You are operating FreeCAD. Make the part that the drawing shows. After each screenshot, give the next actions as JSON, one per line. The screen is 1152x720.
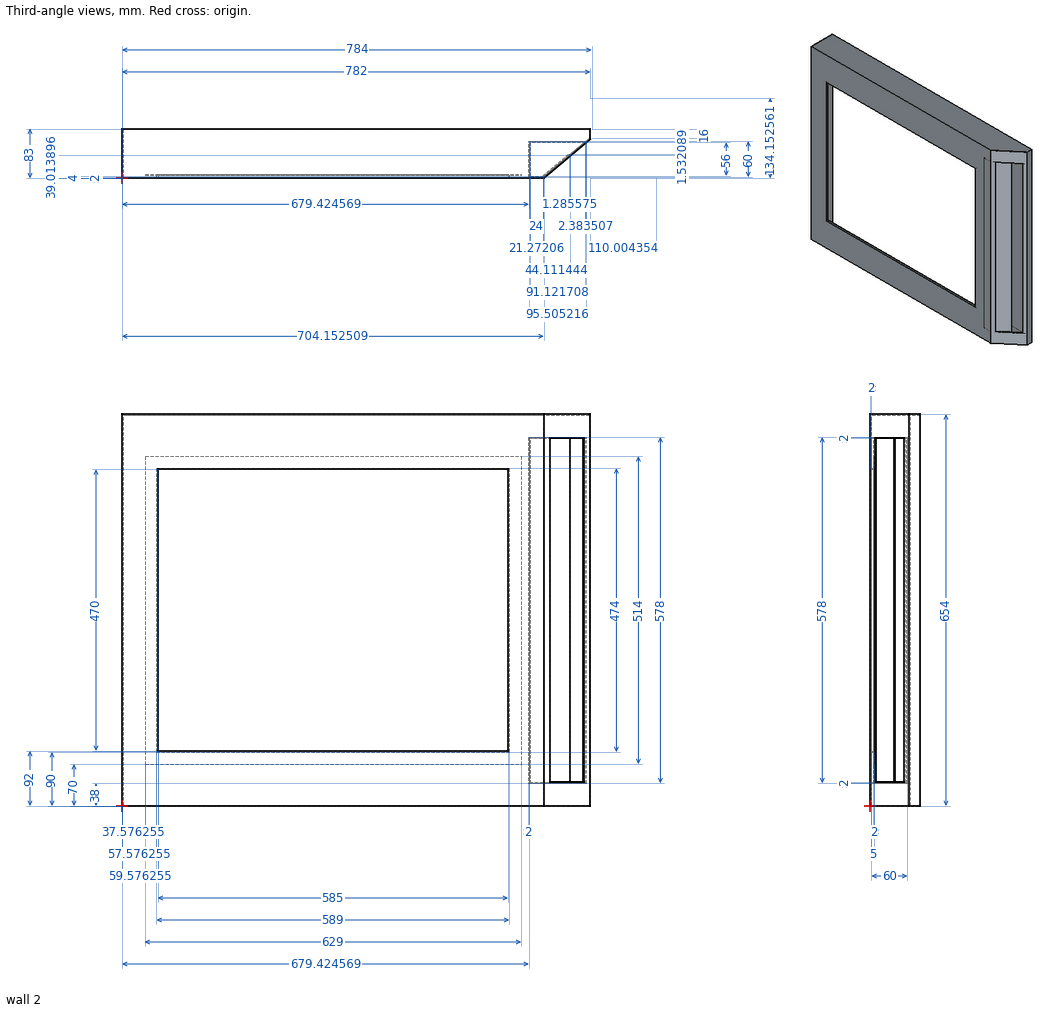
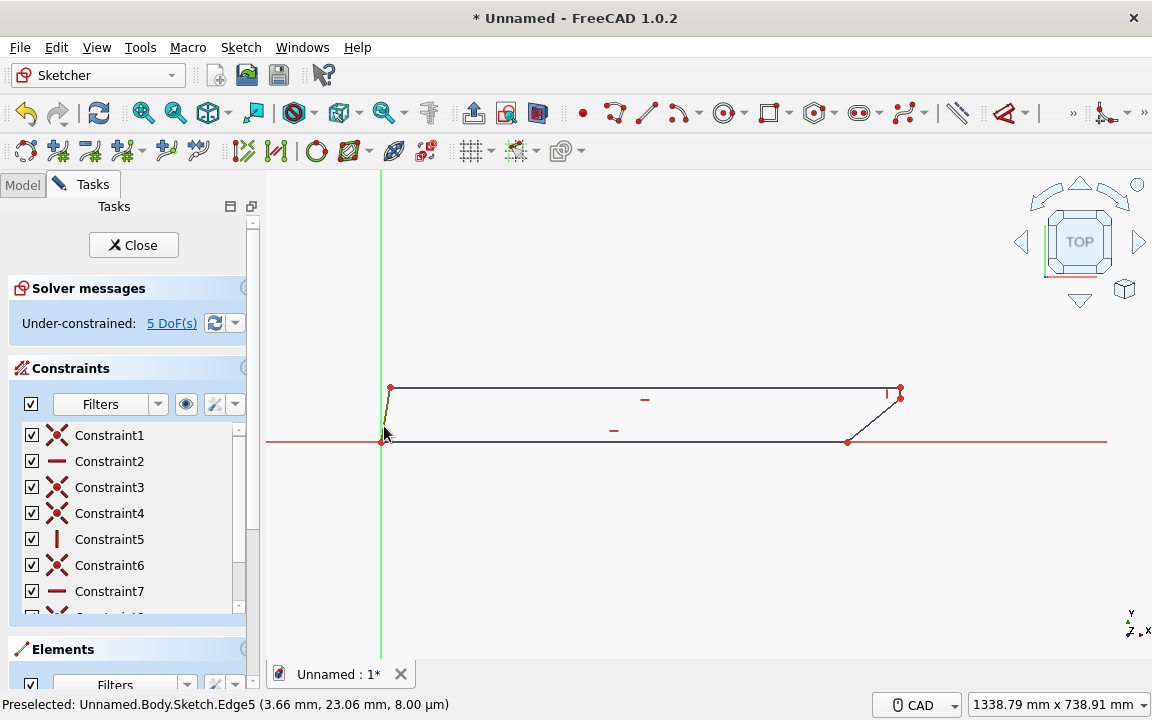
{"action": "key", "text": "v"}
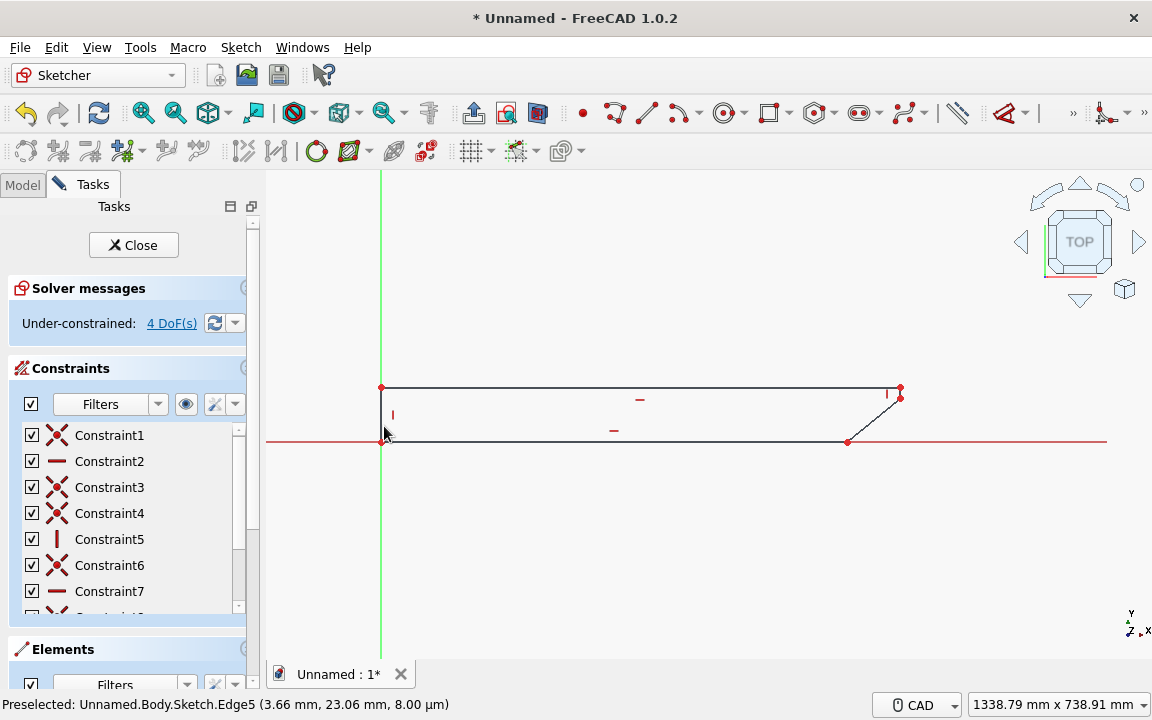
{"action": "key", "text": "d"}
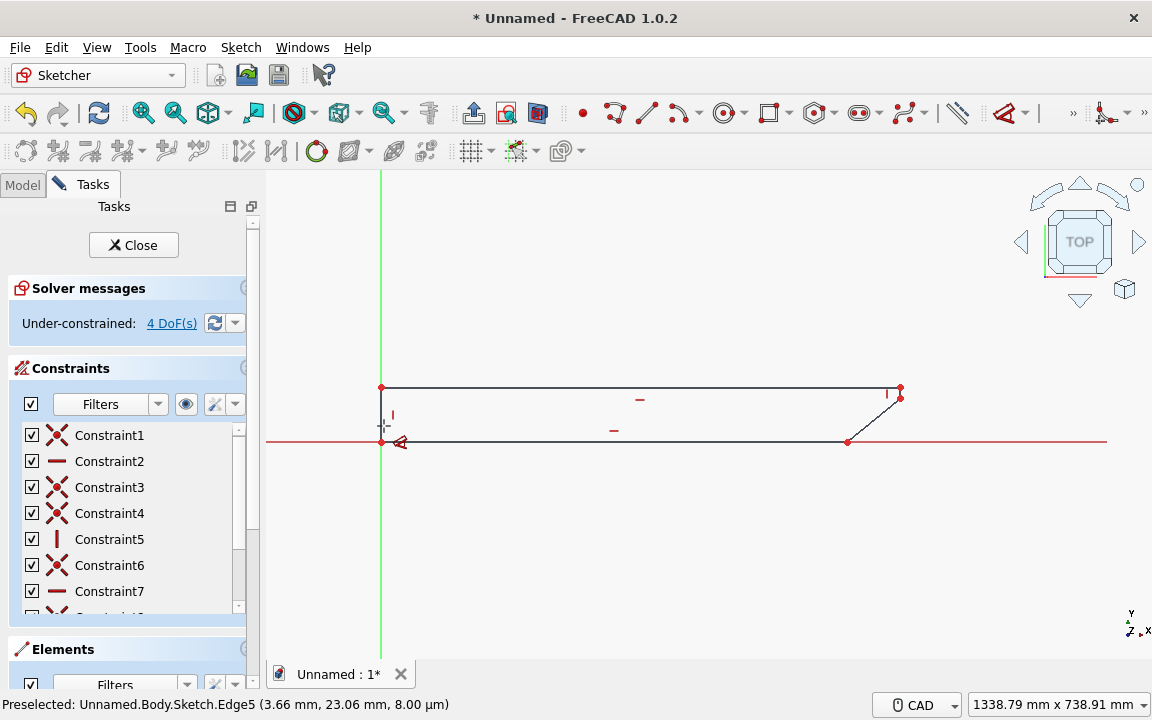
{"action": "scroll", "coordinate": [900, 393], "scroll_direction": "up", "scroll_amount": 7}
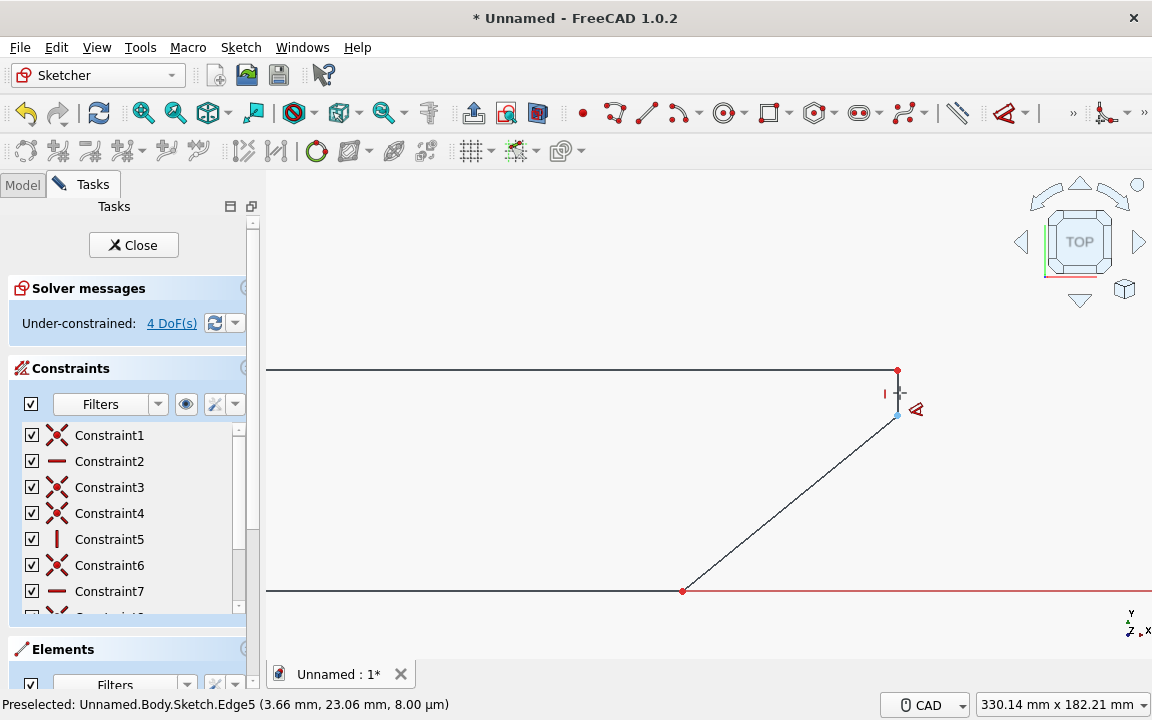
{"action": "left_click", "coordinate": [898, 393]}
{"action": "left_click", "coordinate": [932, 393]}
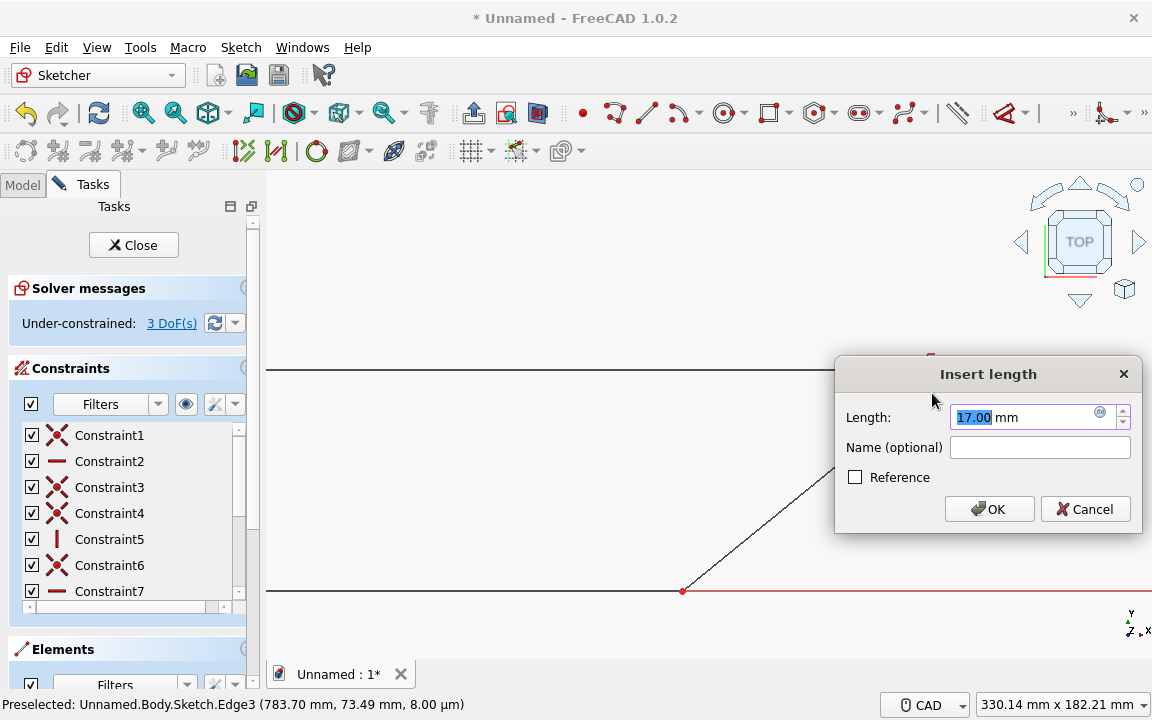
{"action": "type", "text": "16"}
{"action": "key", "text": "Return"}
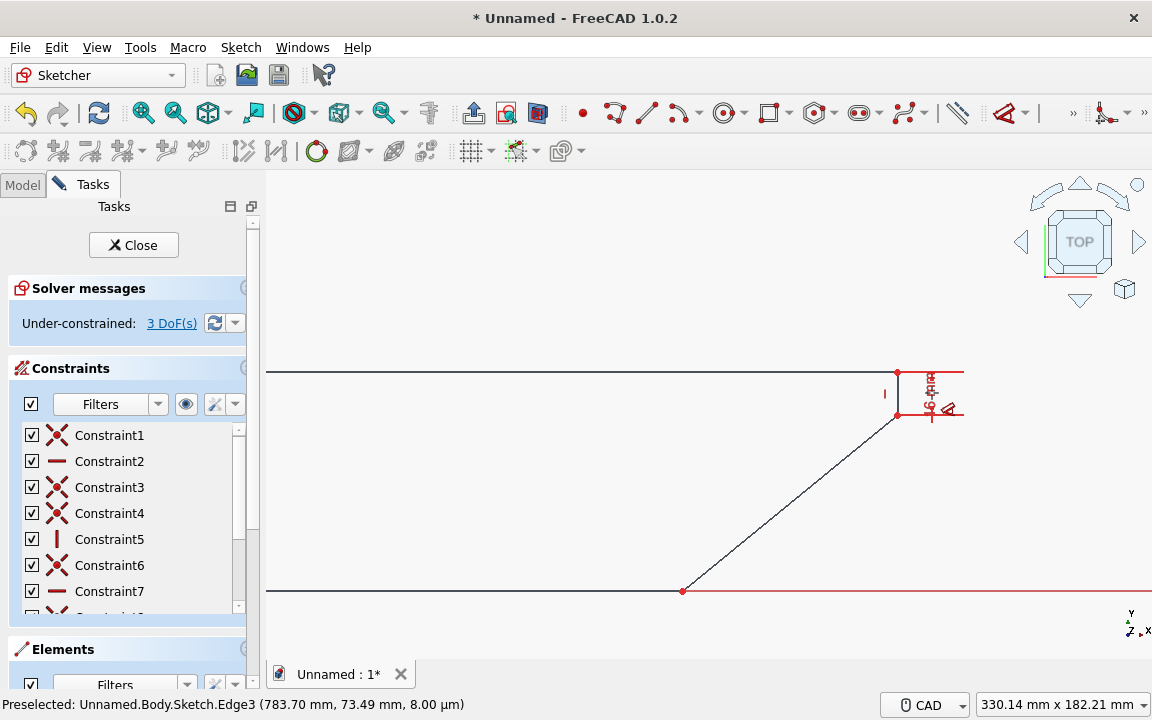
{"action": "scroll", "coordinate": [900, 393], "scroll_direction": "down", "scroll_amount": 7}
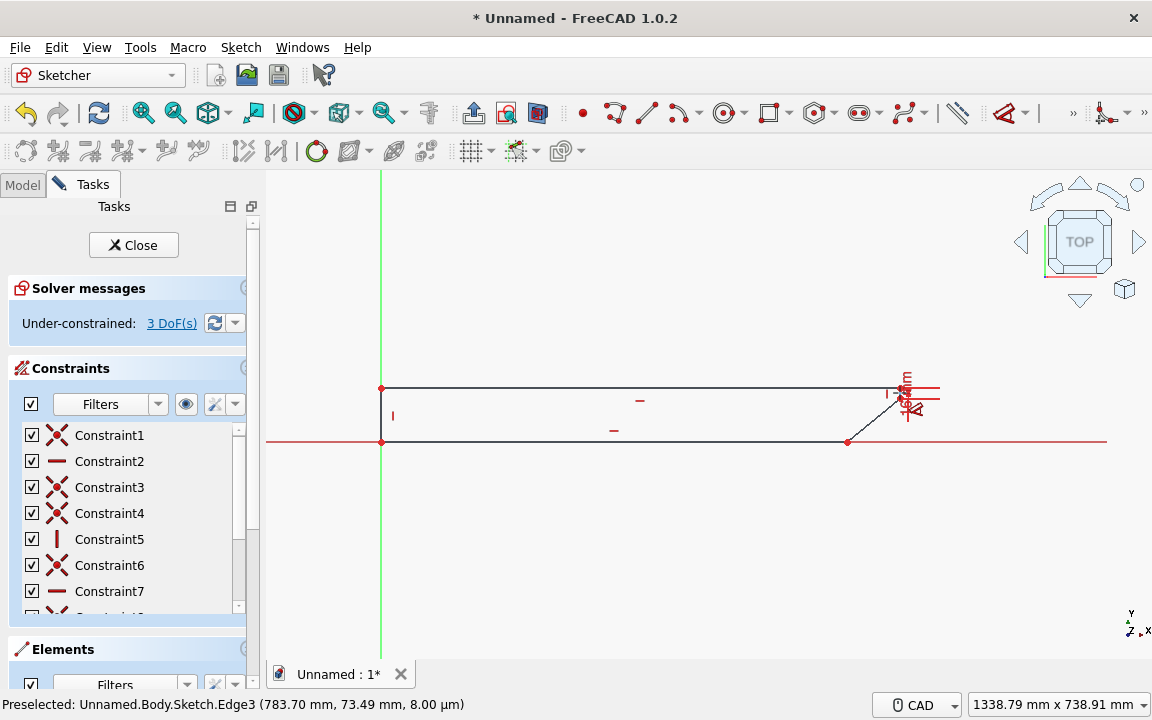
{"action": "left_click", "coordinate": [381, 404]}
{"action": "left_click", "coordinate": [347, 415]}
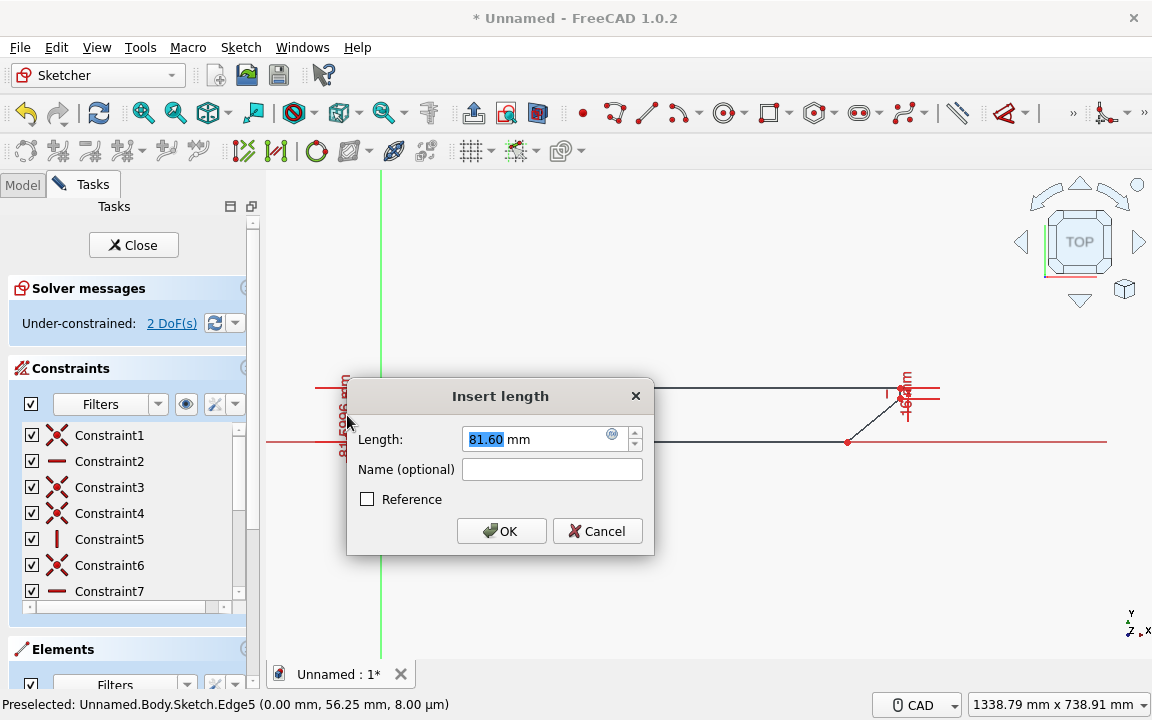
{"action": "type", "text": "83"}
{"action": "key", "text": "Return"}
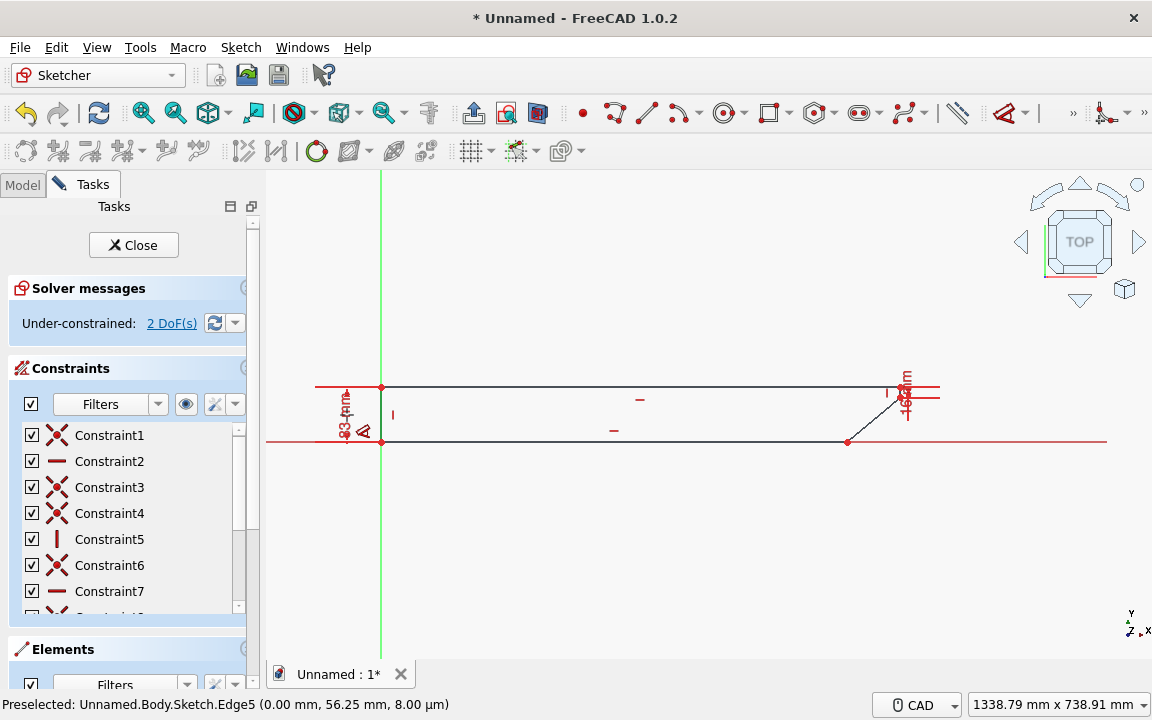
{"action": "left_click", "coordinate": [744, 387]}
{"action": "left_click", "coordinate": [641, 353]}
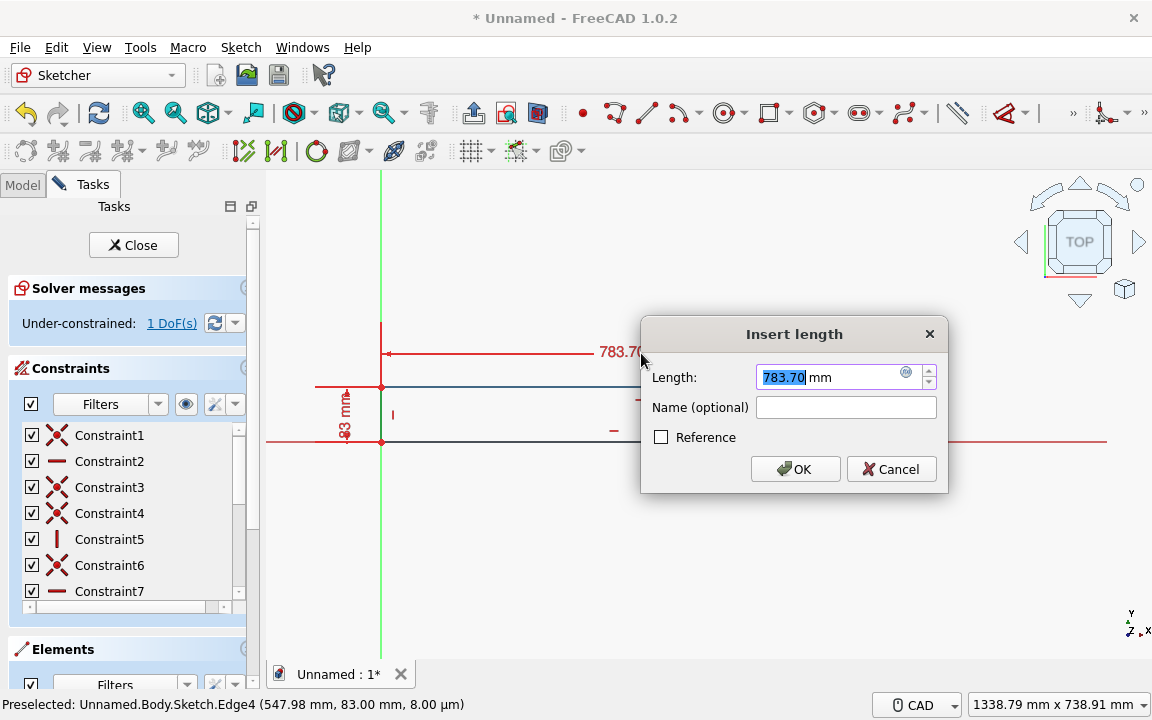
{"action": "type", "text": "784"}
{"action": "key", "text": "Return"}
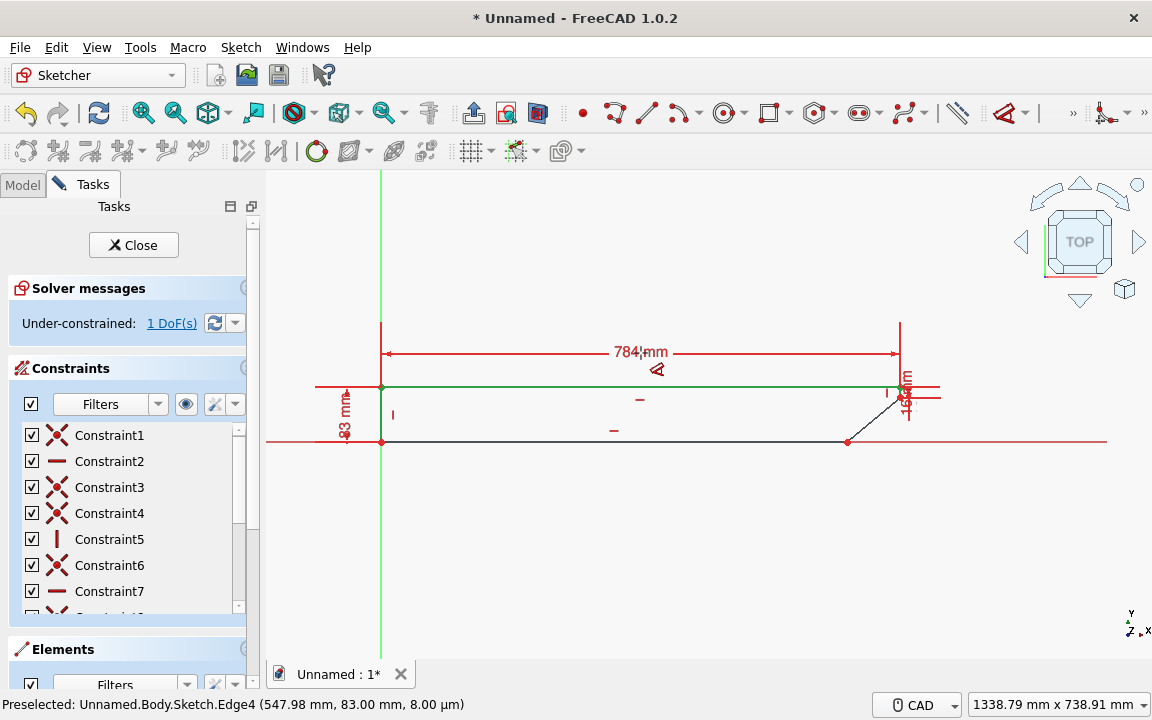
{"action": "left_click", "coordinate": [521, 442]}
{"action": "left_click", "coordinate": [614, 476]}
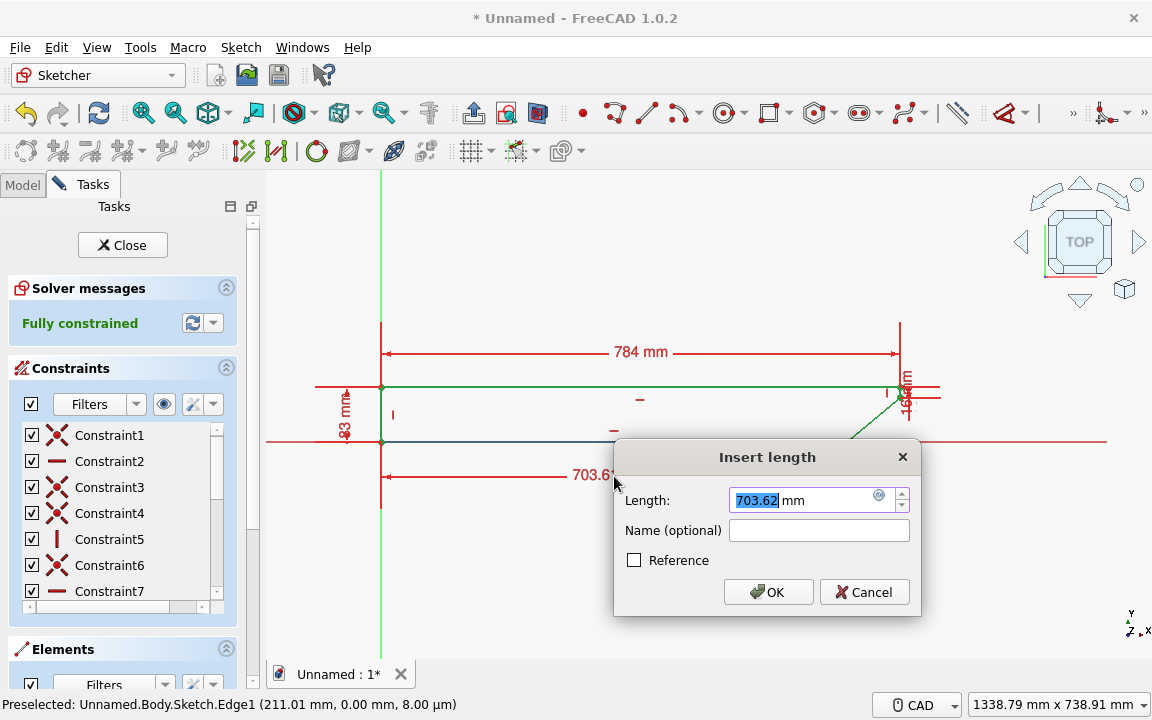
{"action": "type", "text": "704.152509"}
{"action": "key", "text": "Return"}
{"action": "key", "text": "Escape"}